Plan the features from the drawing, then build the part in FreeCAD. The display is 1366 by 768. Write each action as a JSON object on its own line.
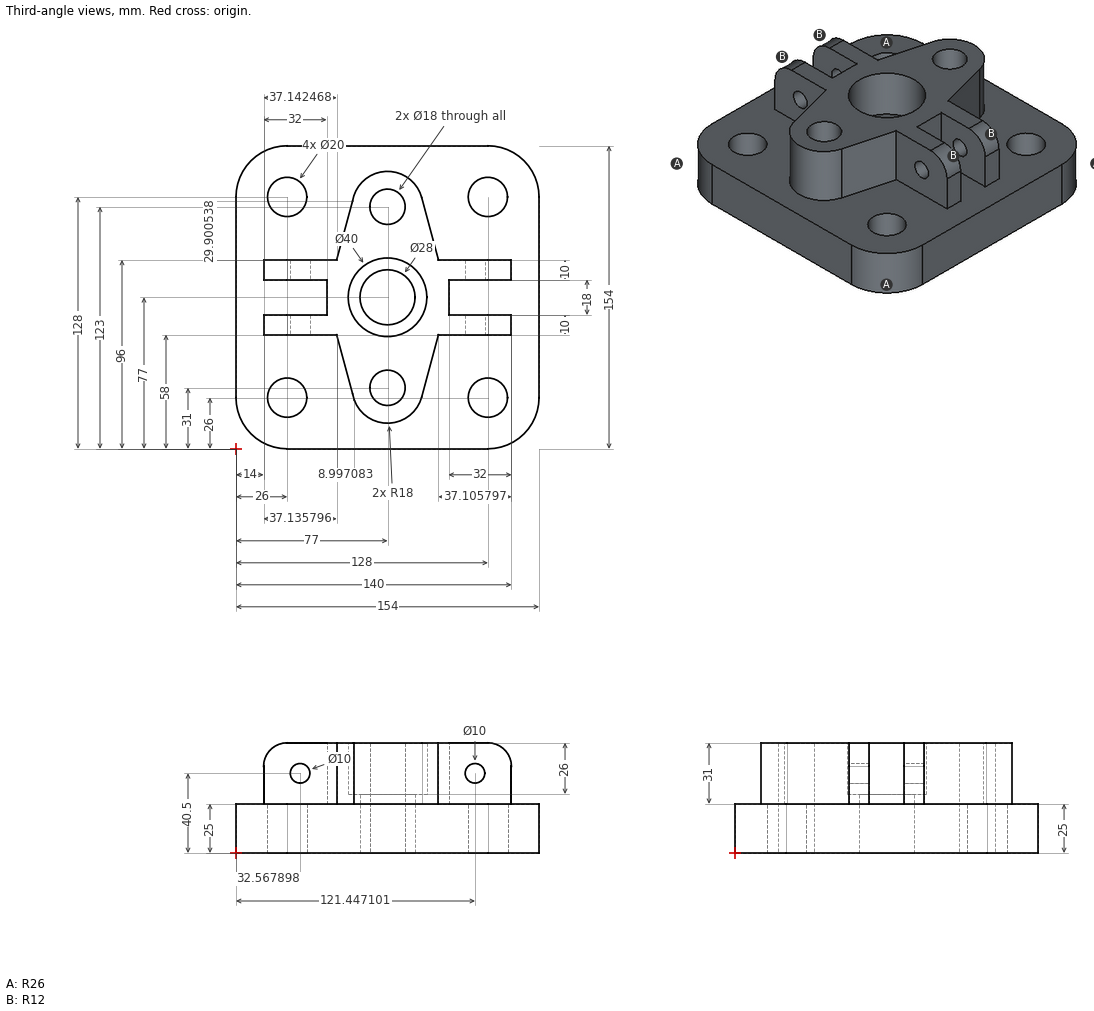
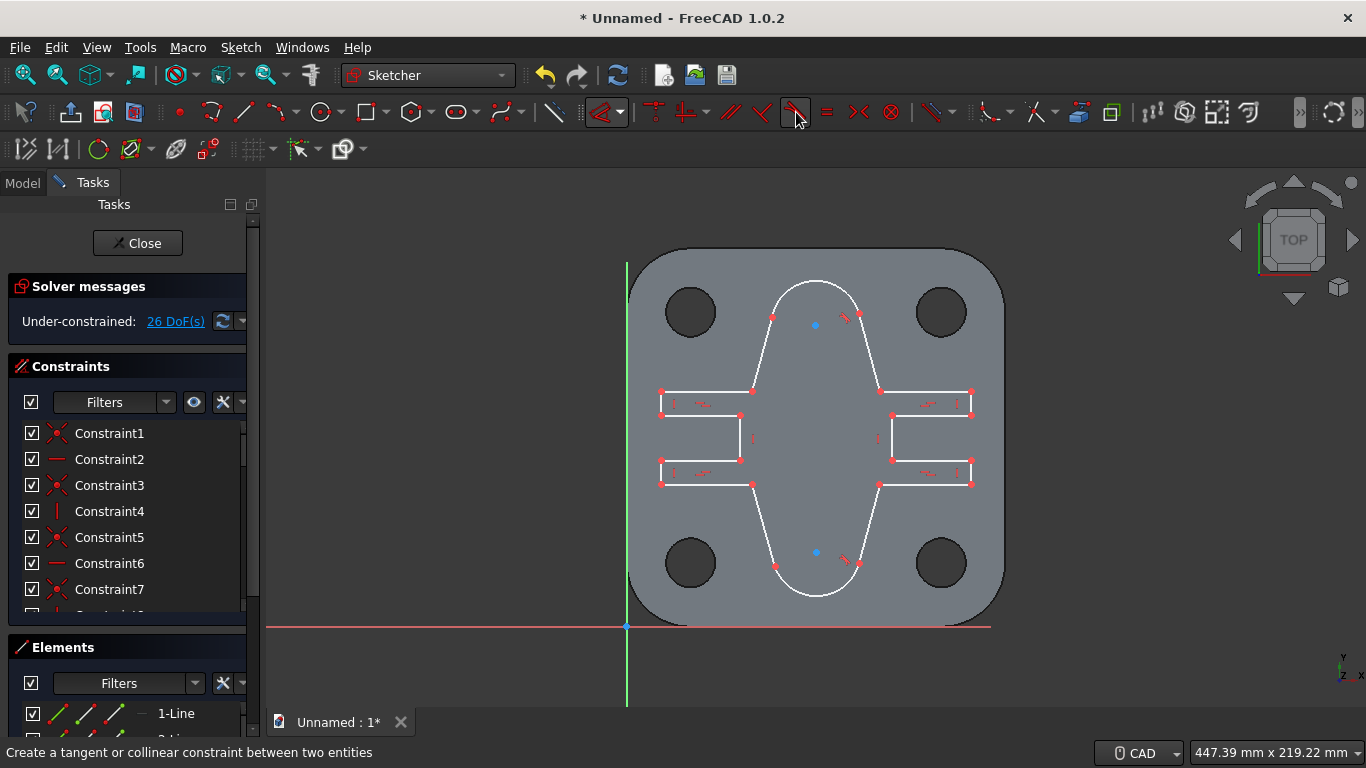
{"action": "left_click", "coordinate": [837, 286]}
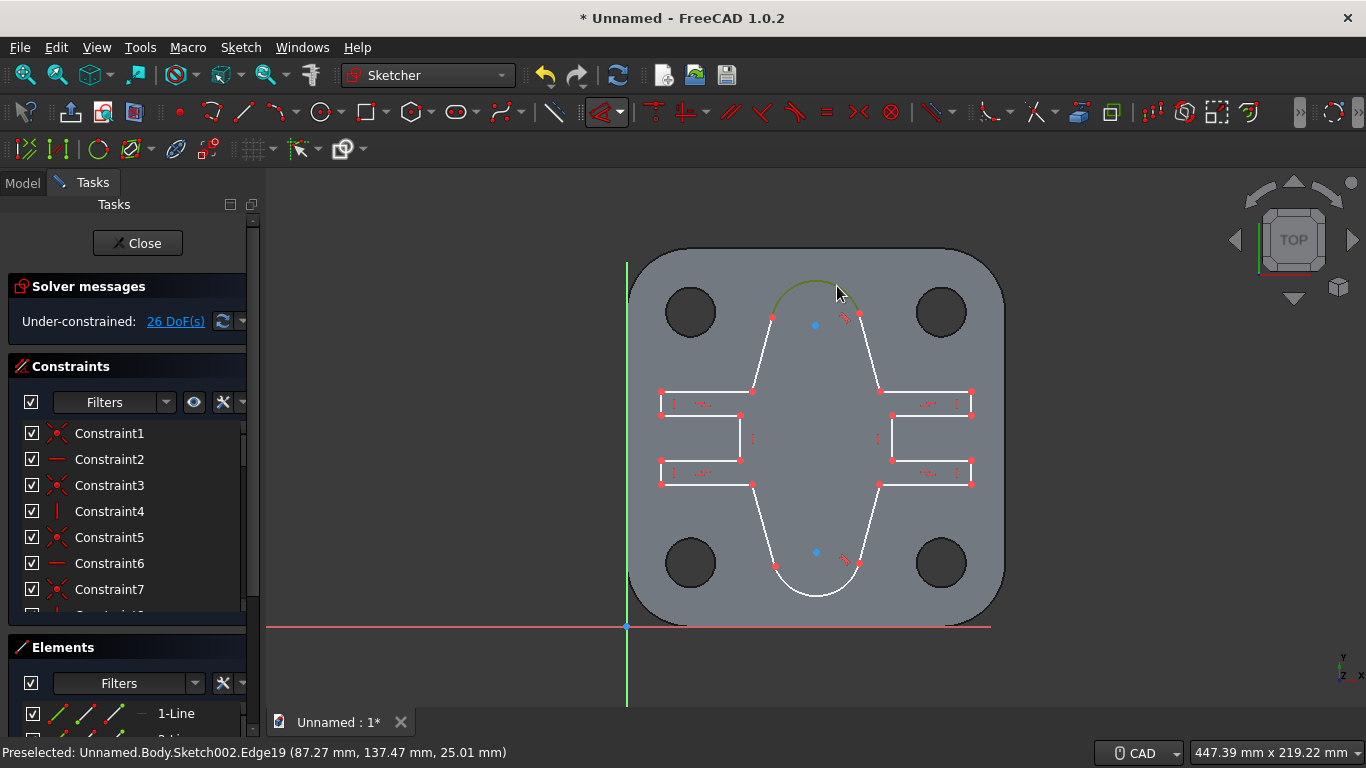
{"action": "left_click", "coordinate": [797, 591]}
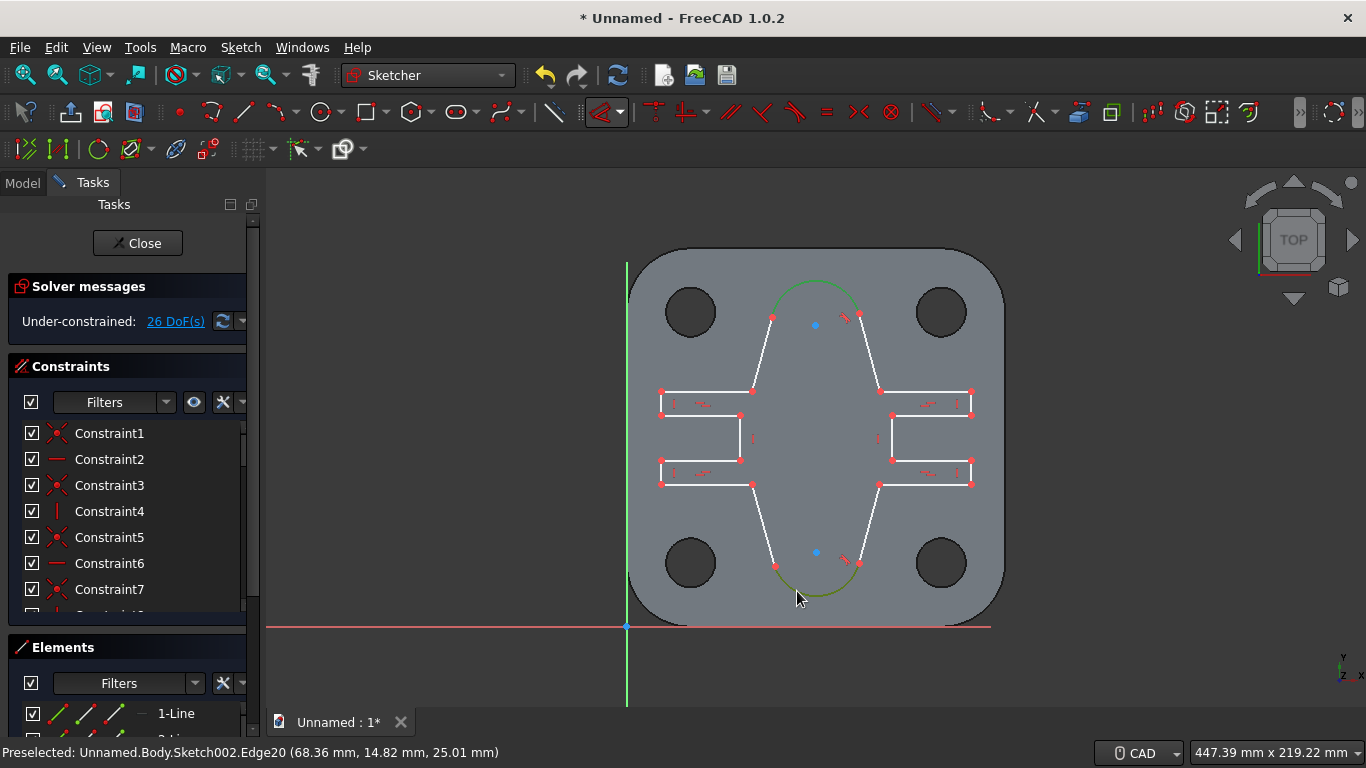
{"action": "left_click", "coordinate": [828, 112]}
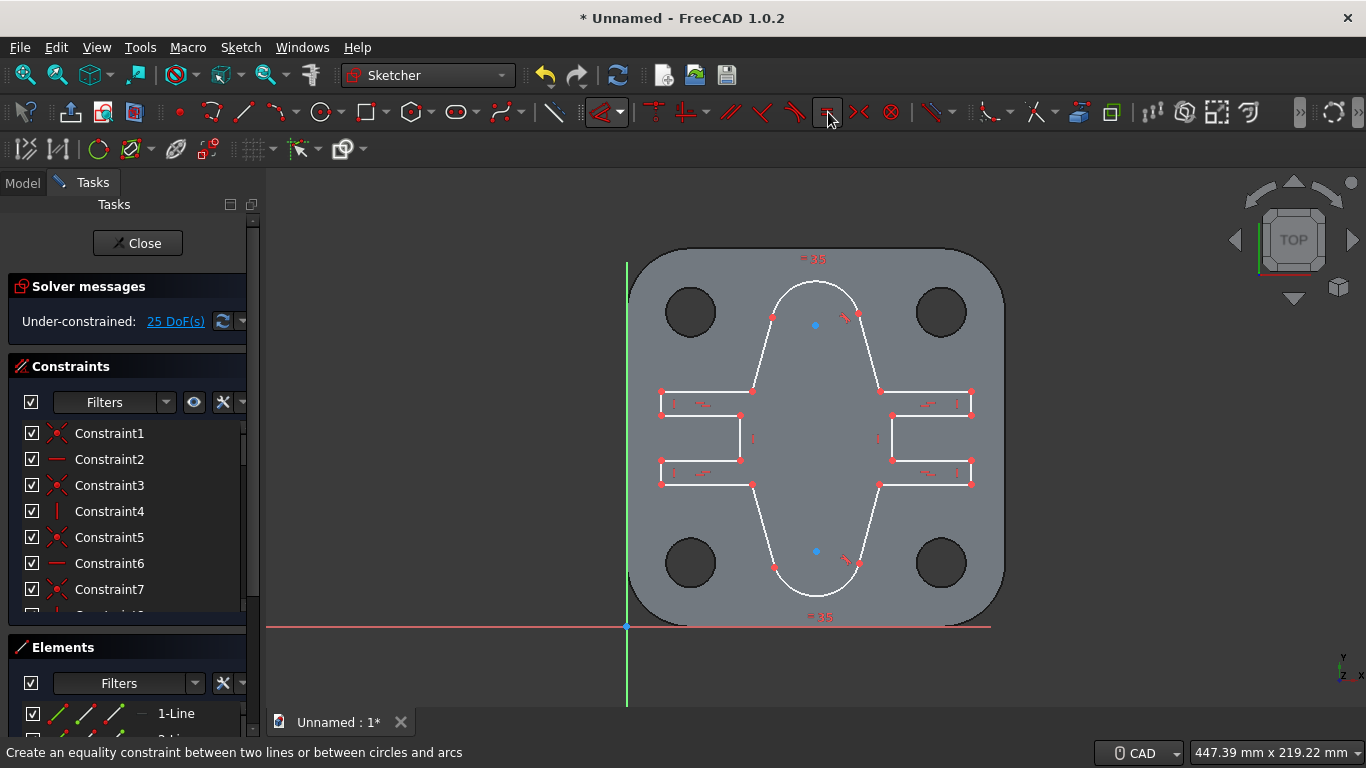
{"action": "left_click", "coordinate": [837, 287]}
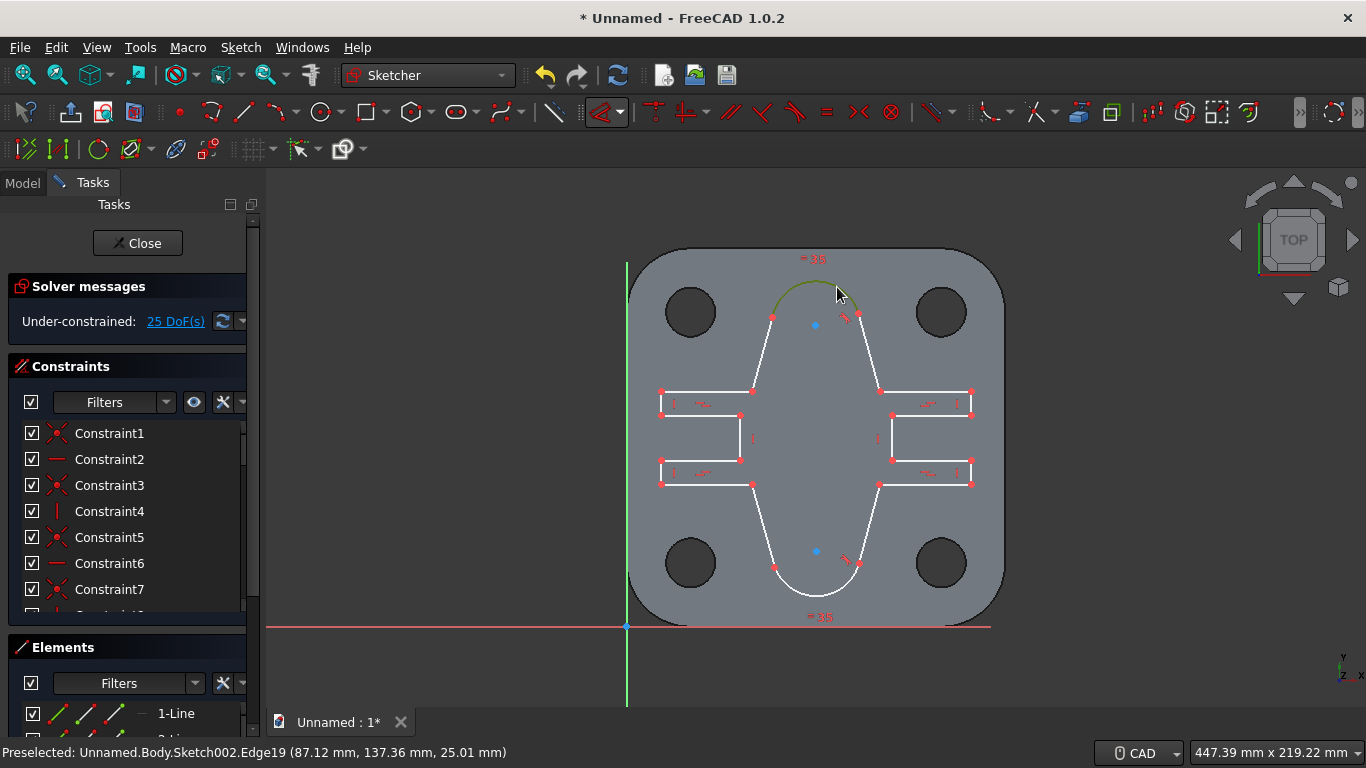
{"action": "left_click", "coordinate": [622, 112]}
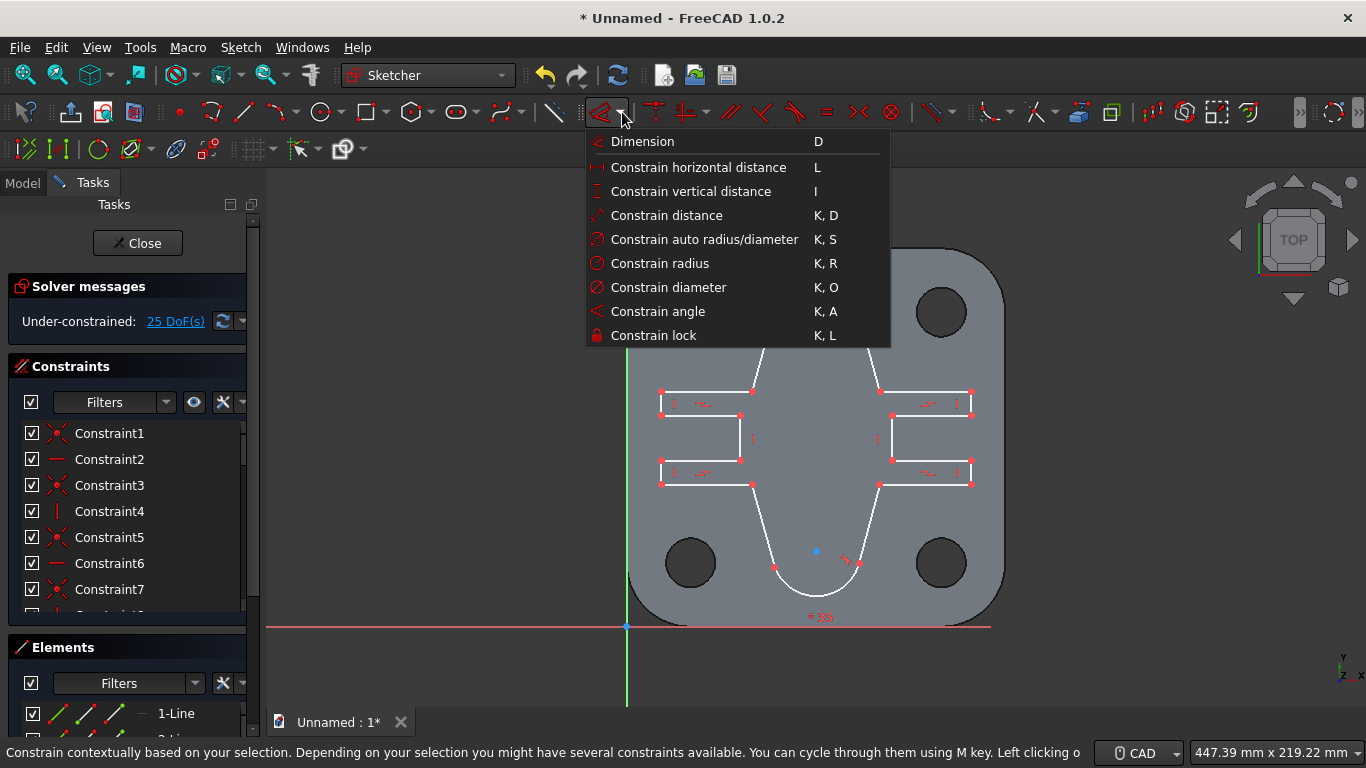
{"action": "left_click", "coordinate": [738, 263]}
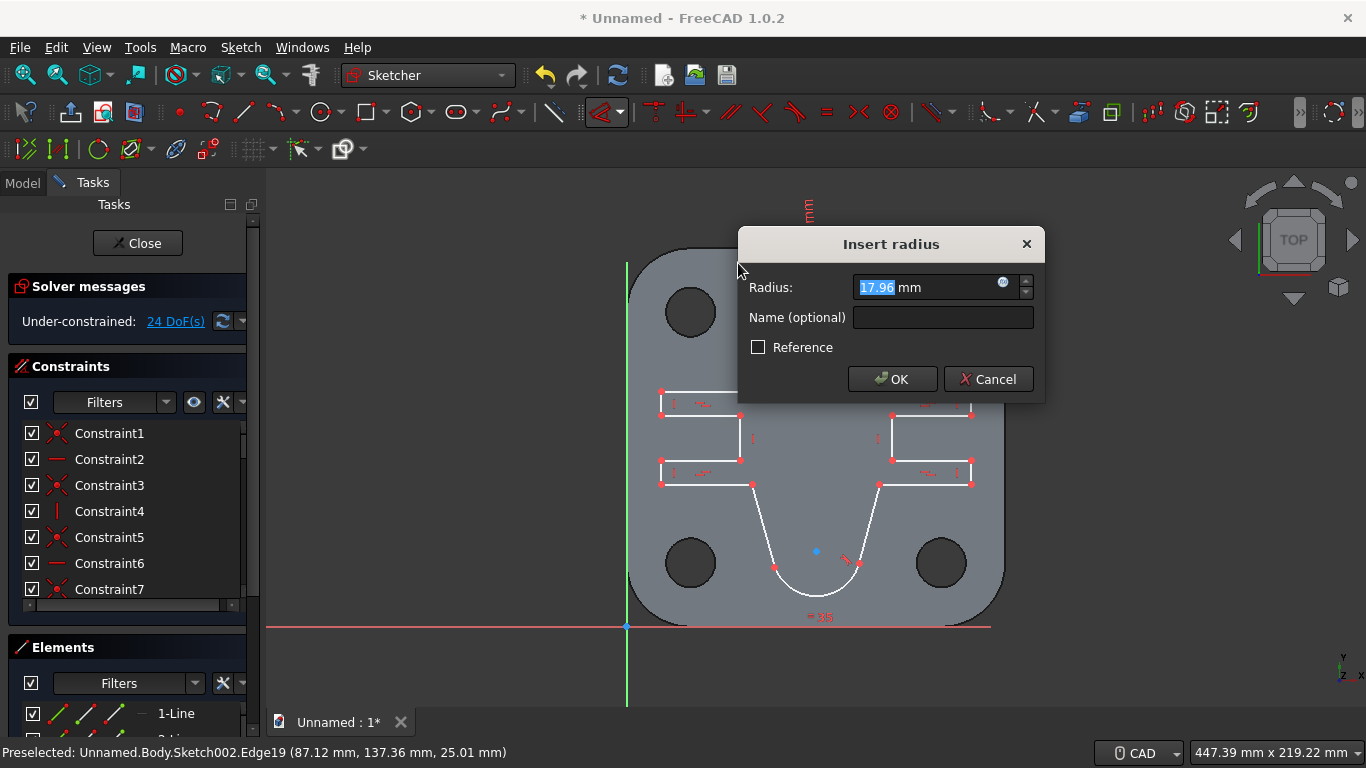
{"action": "type", "text": "18"}
{"action": "key", "text": "Return"}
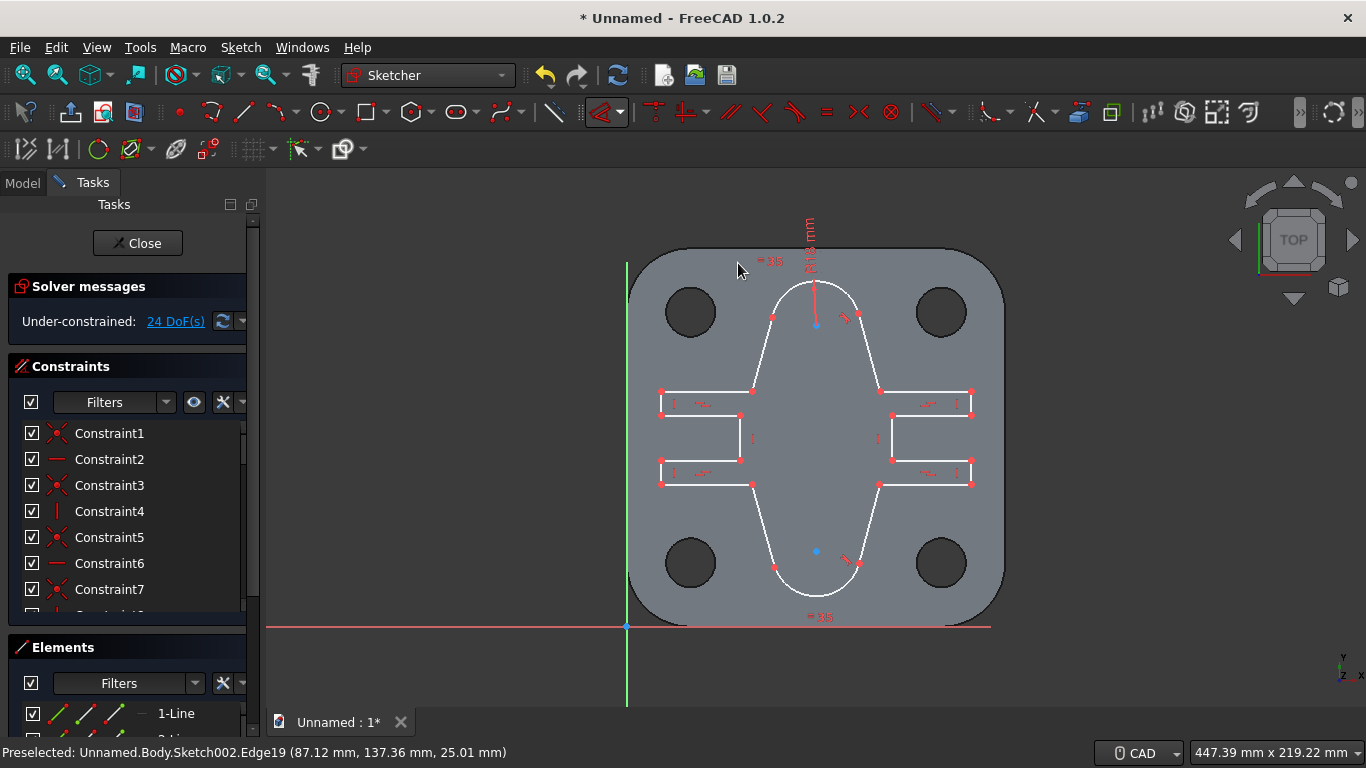
{"action": "scroll", "coordinate": [971, 475], "scroll_direction": "up", "scroll_amount": 3}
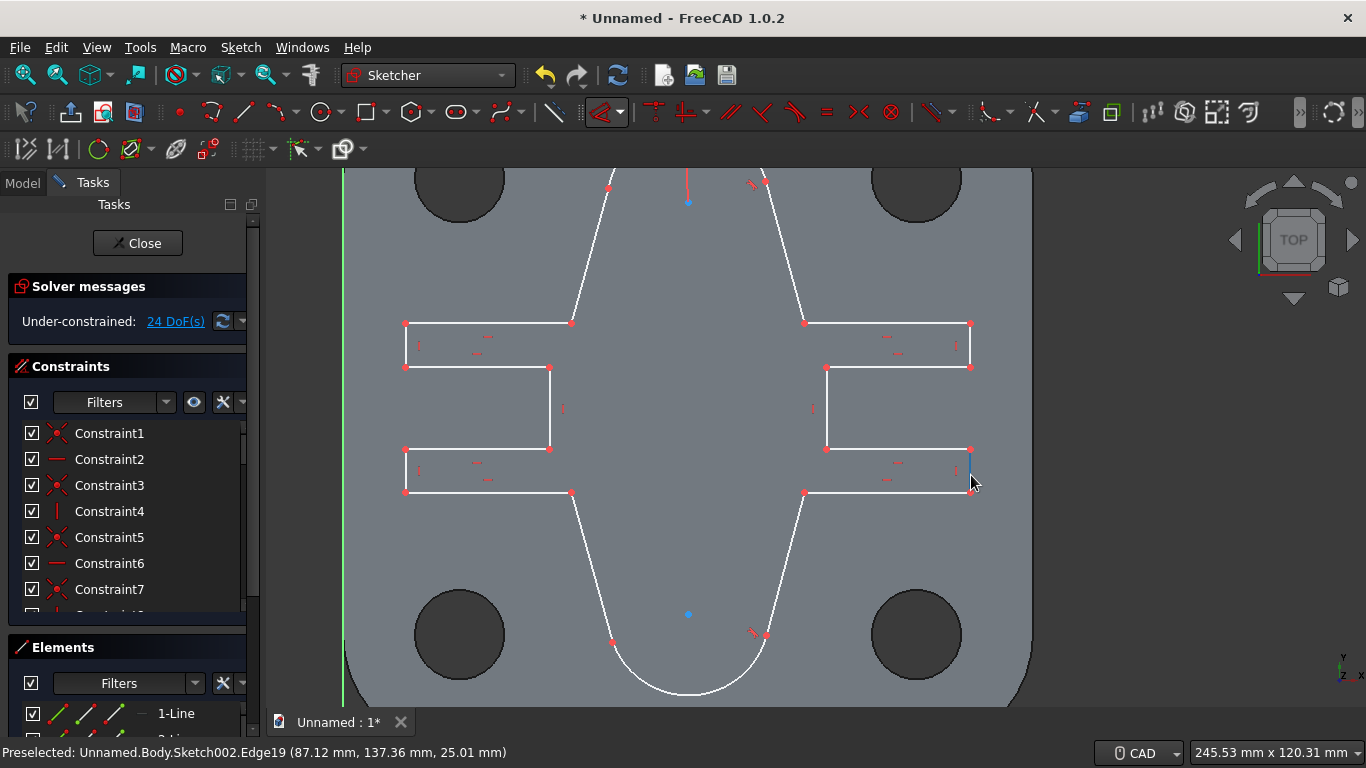
{"action": "left_click", "coordinate": [970, 475]}